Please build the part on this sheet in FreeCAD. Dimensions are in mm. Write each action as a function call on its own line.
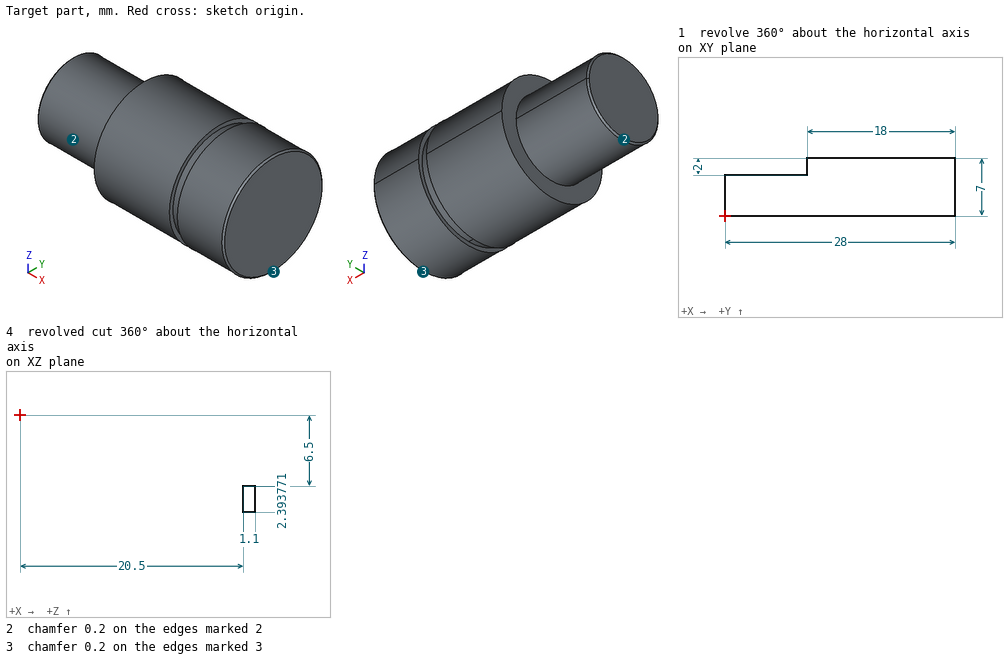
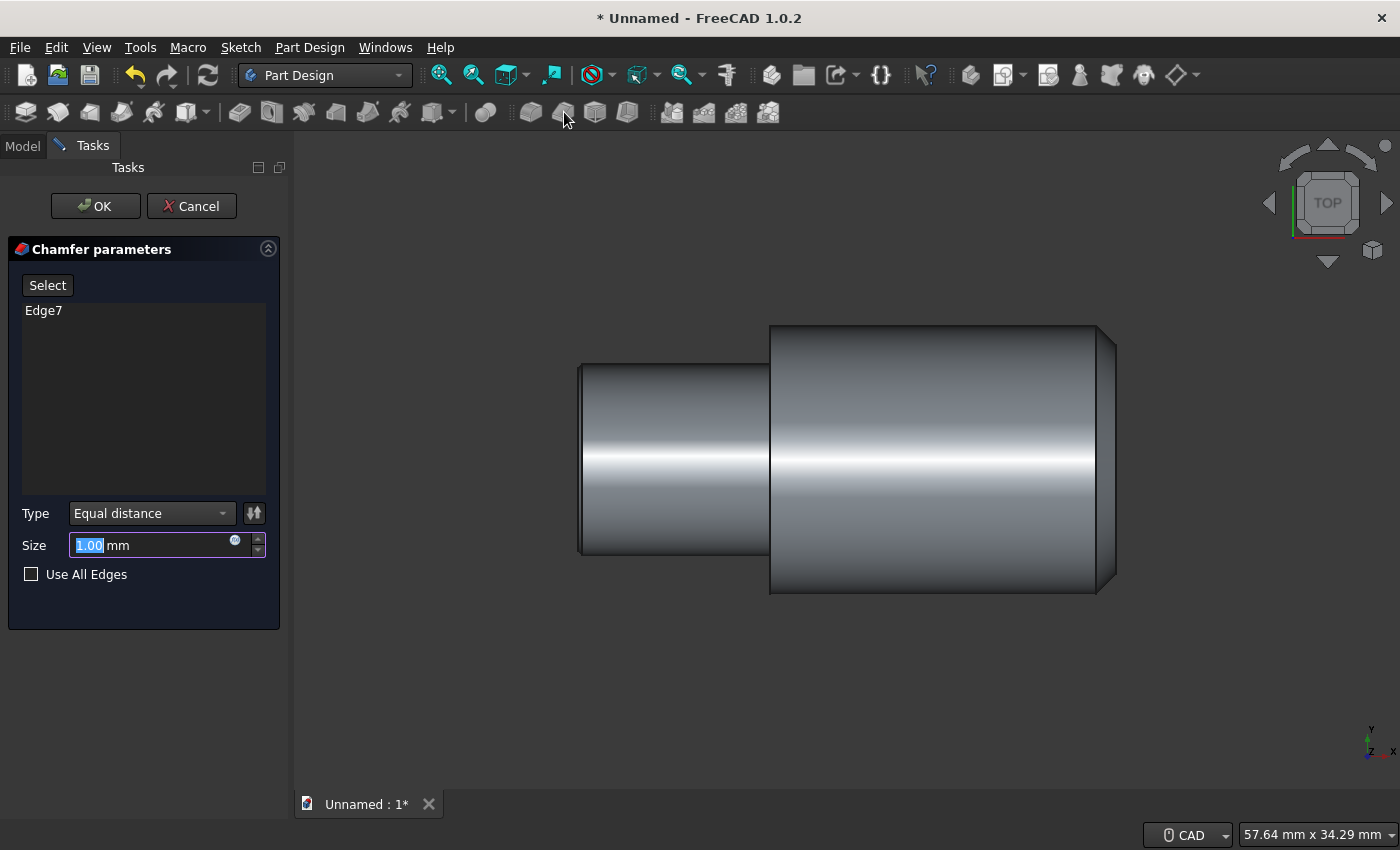
text(0.2)
key(Tab)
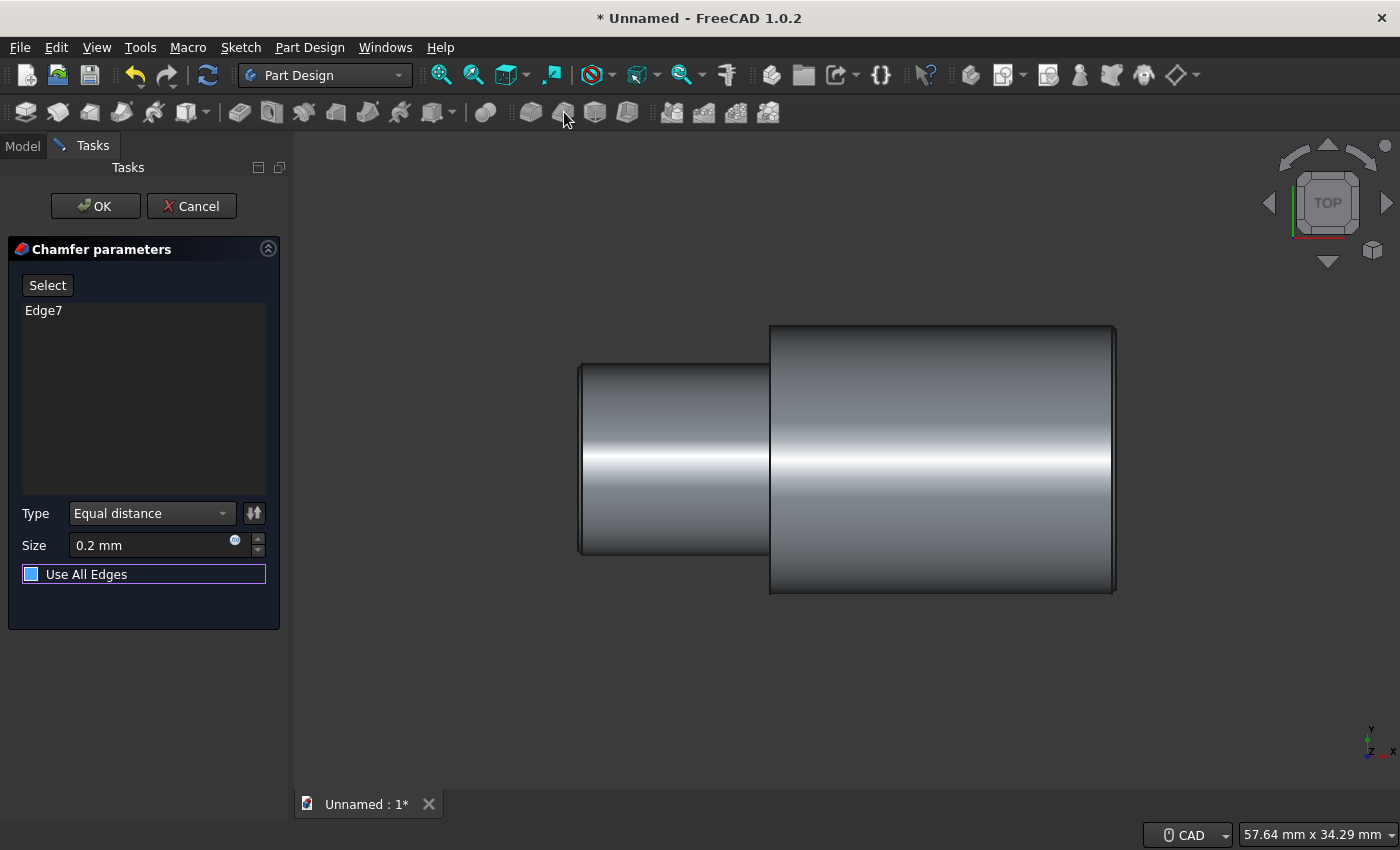
click(96, 206)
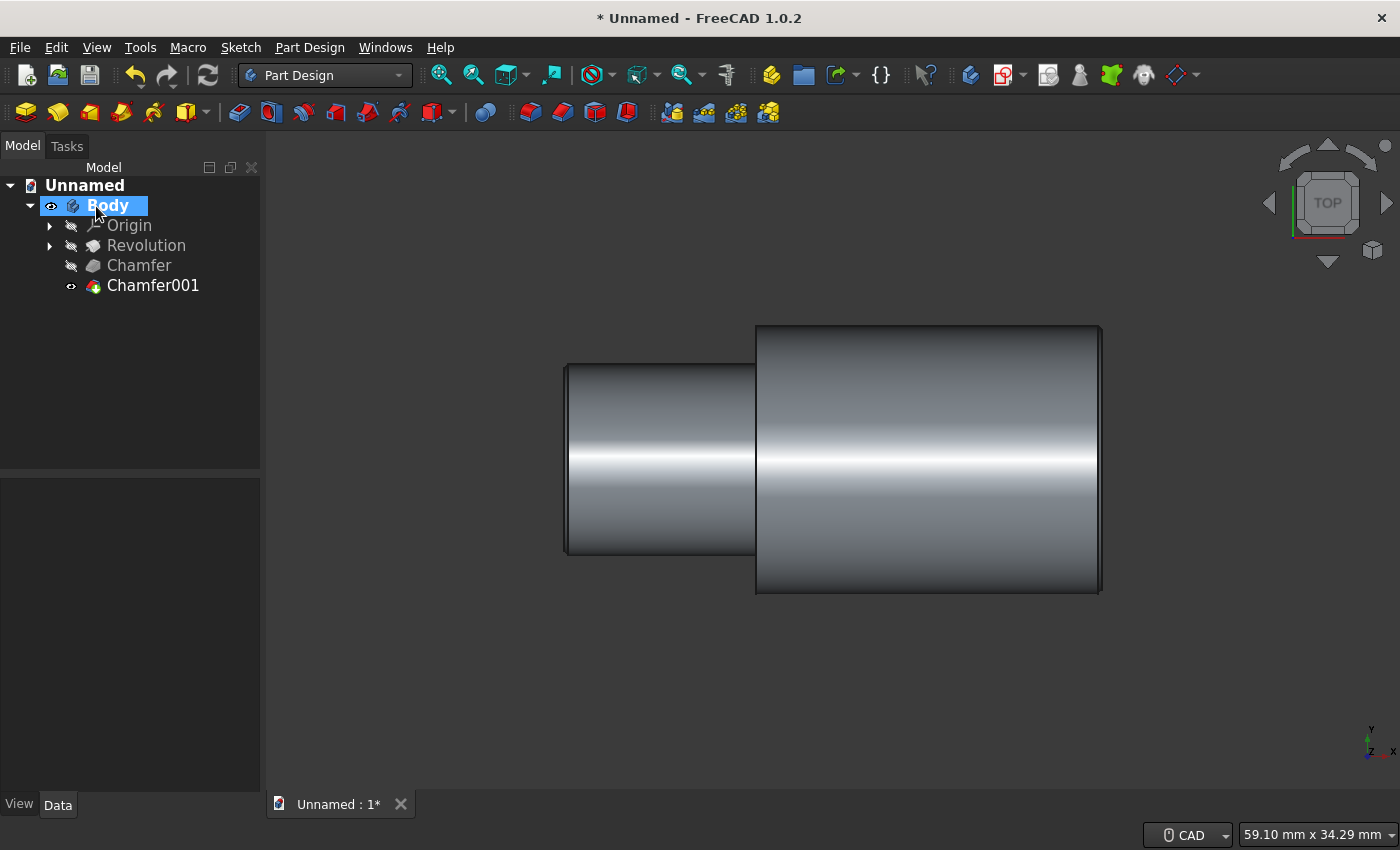
click(1004, 76)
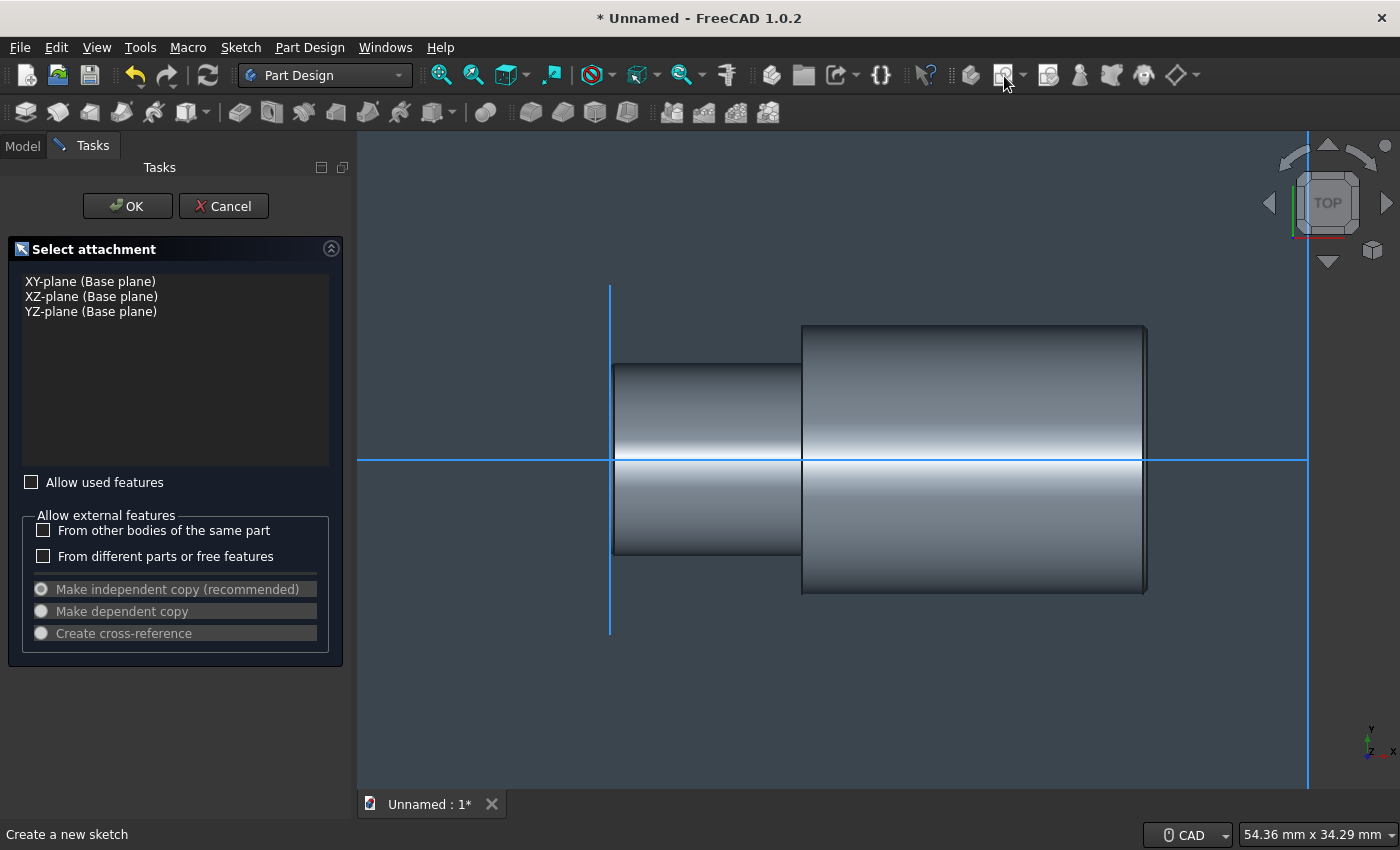
click(82, 296)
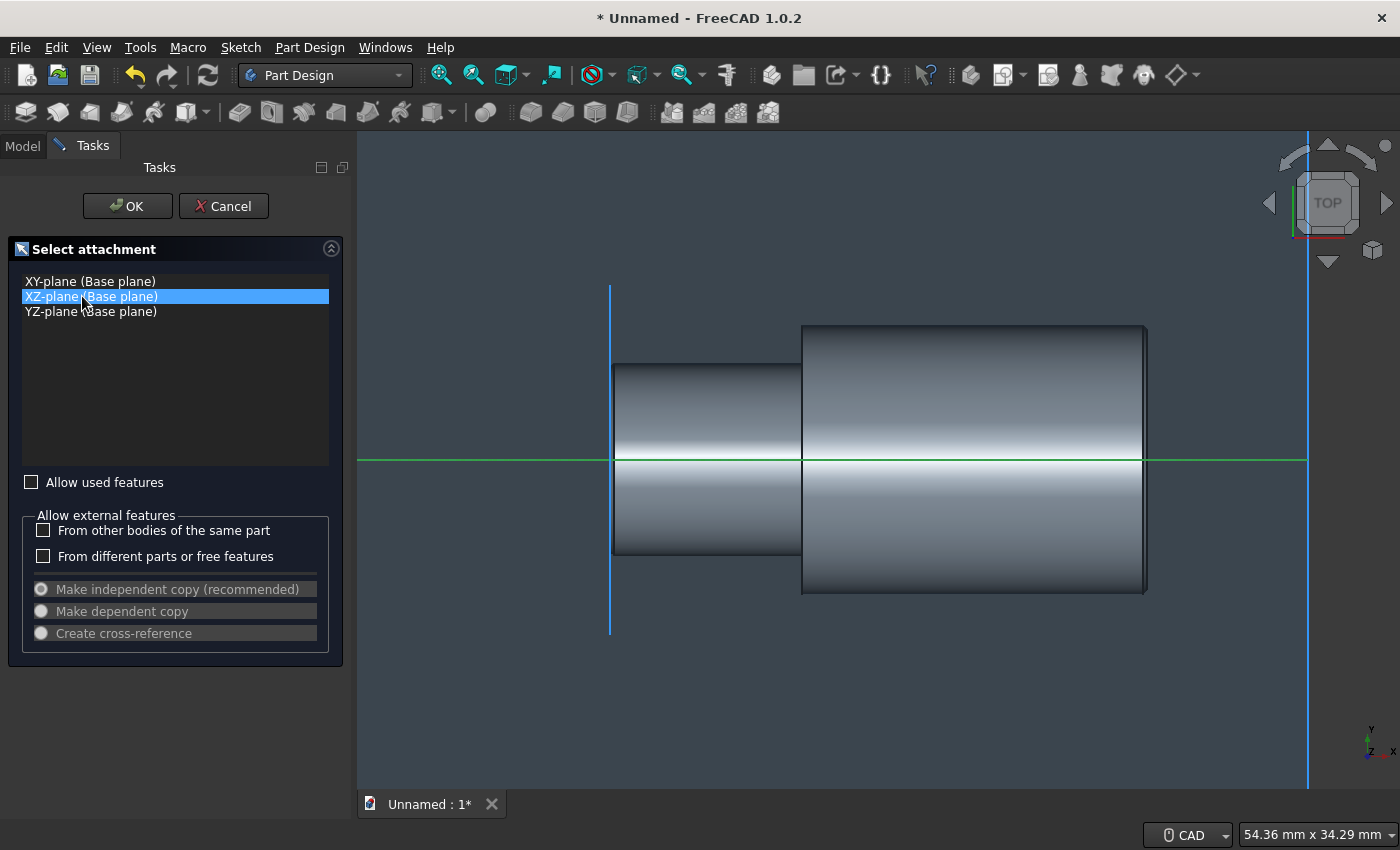
click(128, 206)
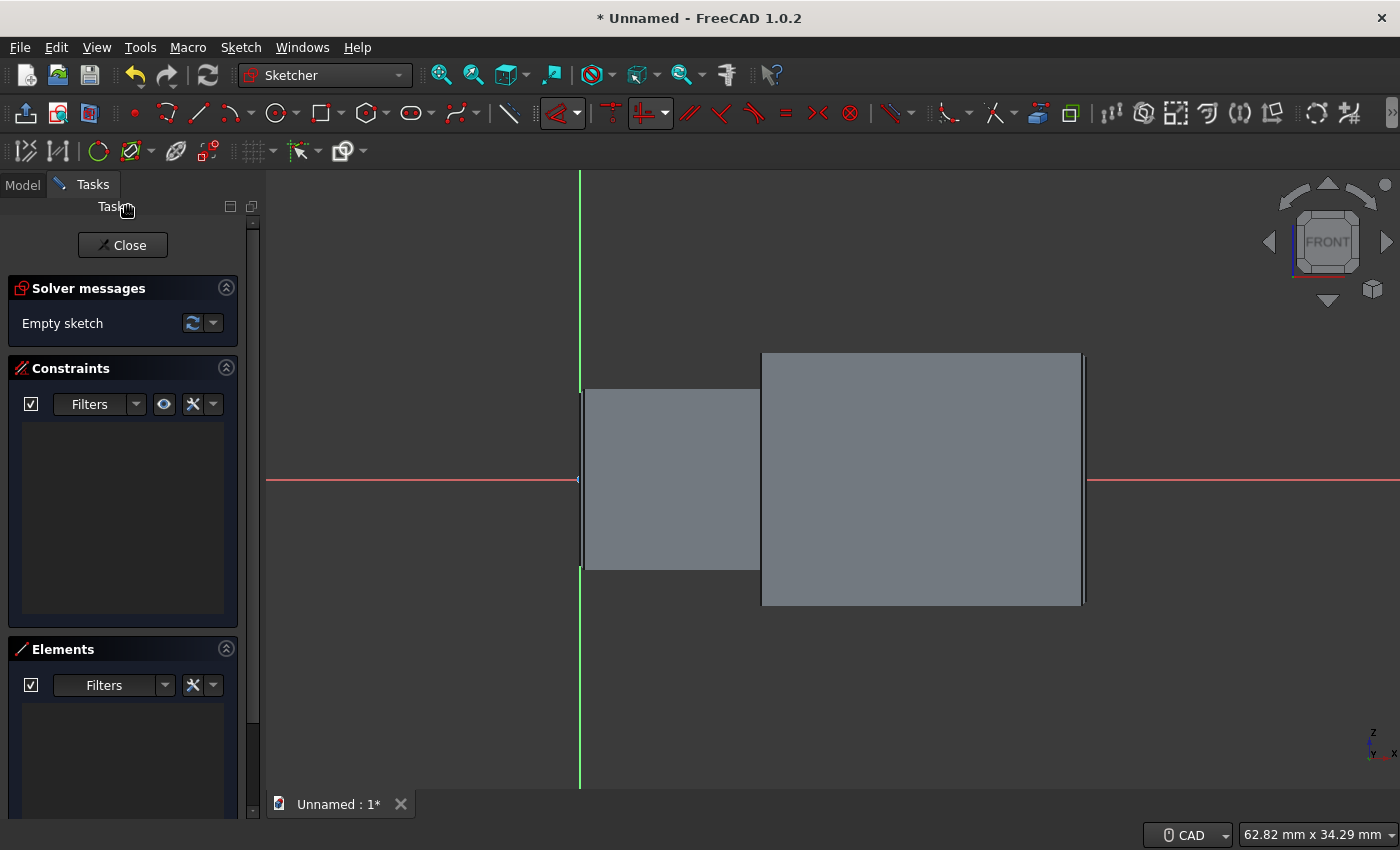
click(90, 114)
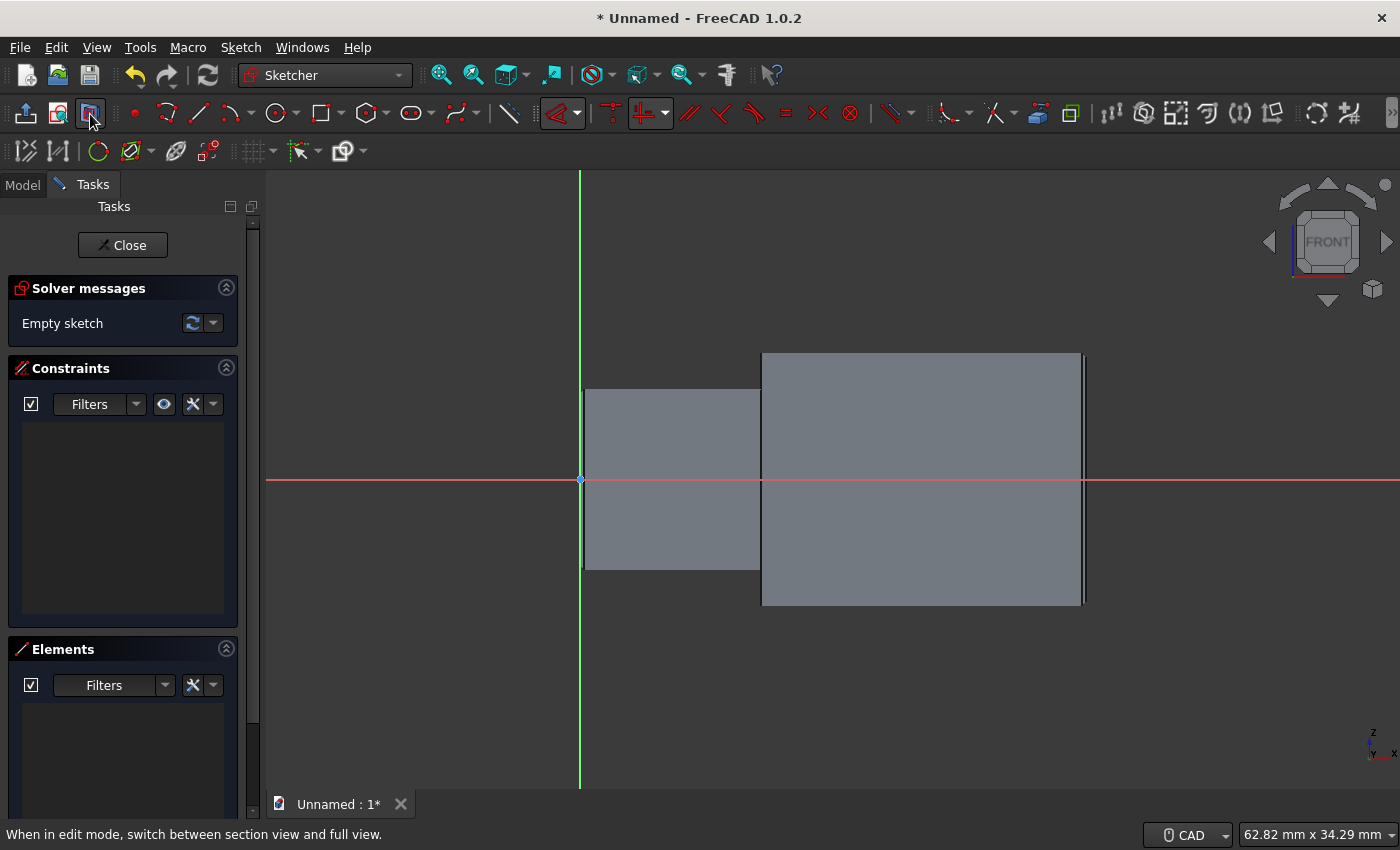
scroll(985, 636, up, 11)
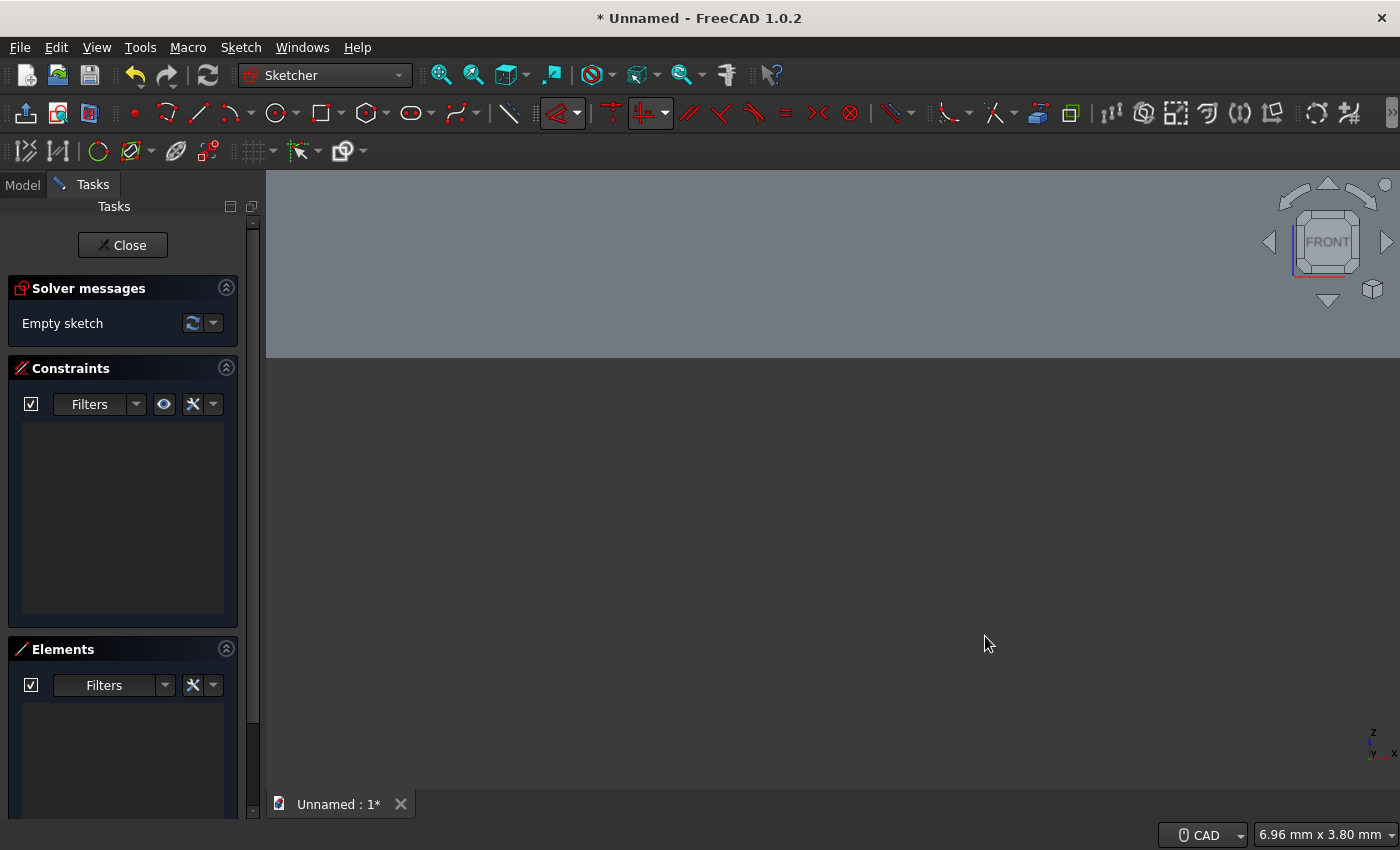
click(322, 114)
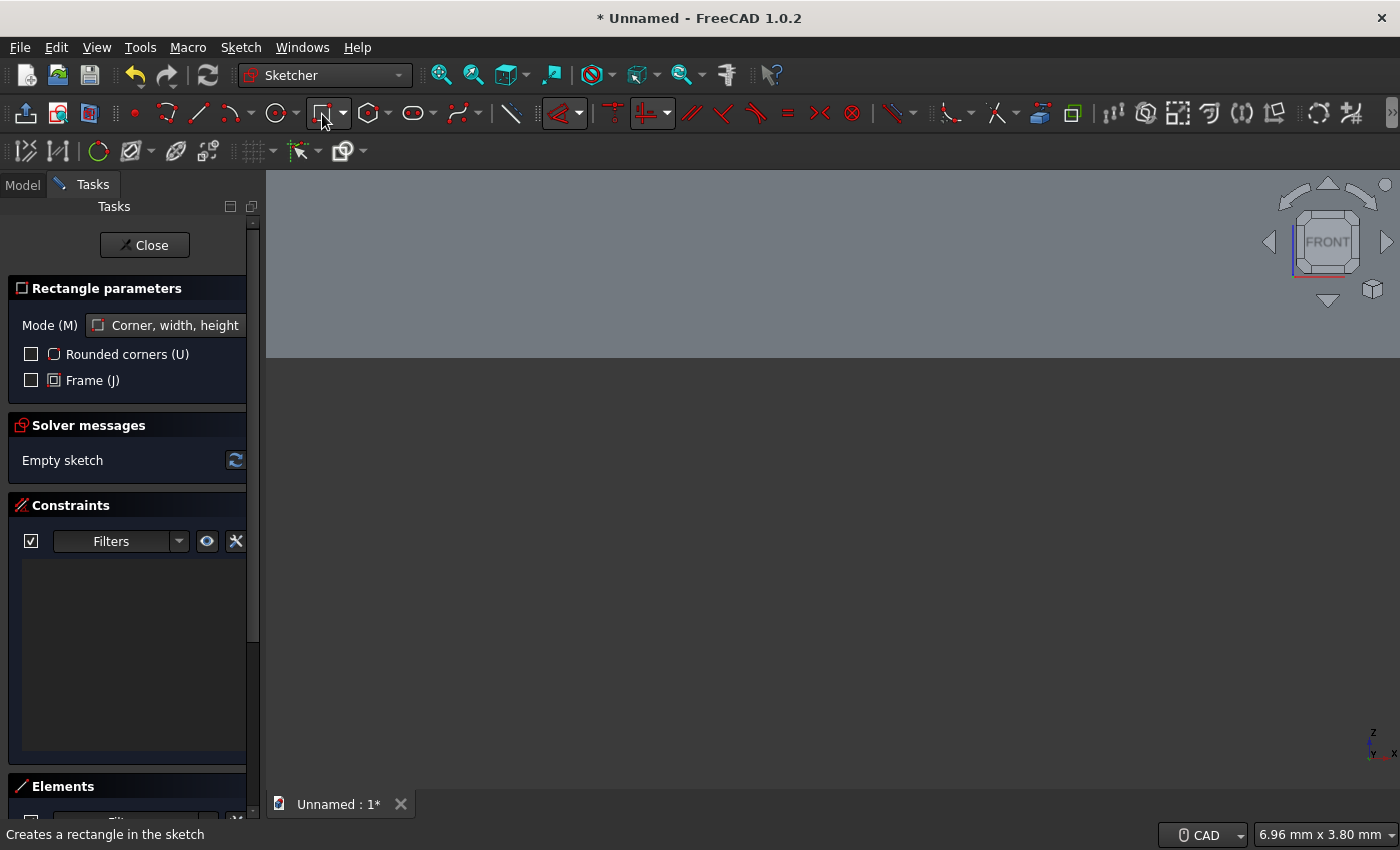
click(667, 276)
click(846, 666)
key(Escape)